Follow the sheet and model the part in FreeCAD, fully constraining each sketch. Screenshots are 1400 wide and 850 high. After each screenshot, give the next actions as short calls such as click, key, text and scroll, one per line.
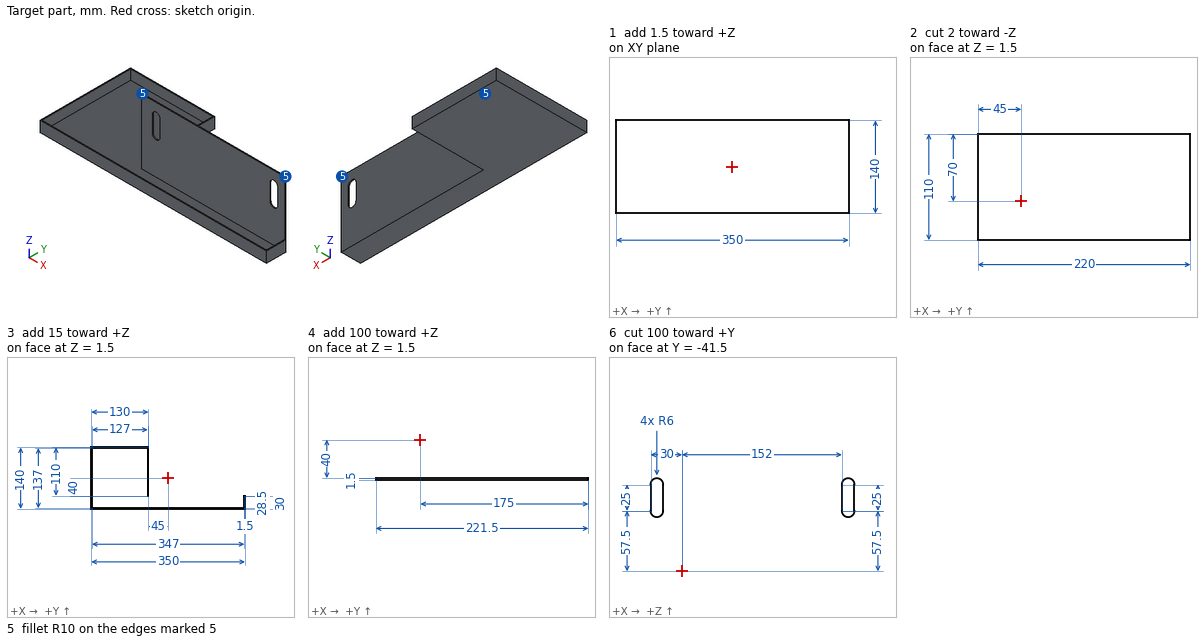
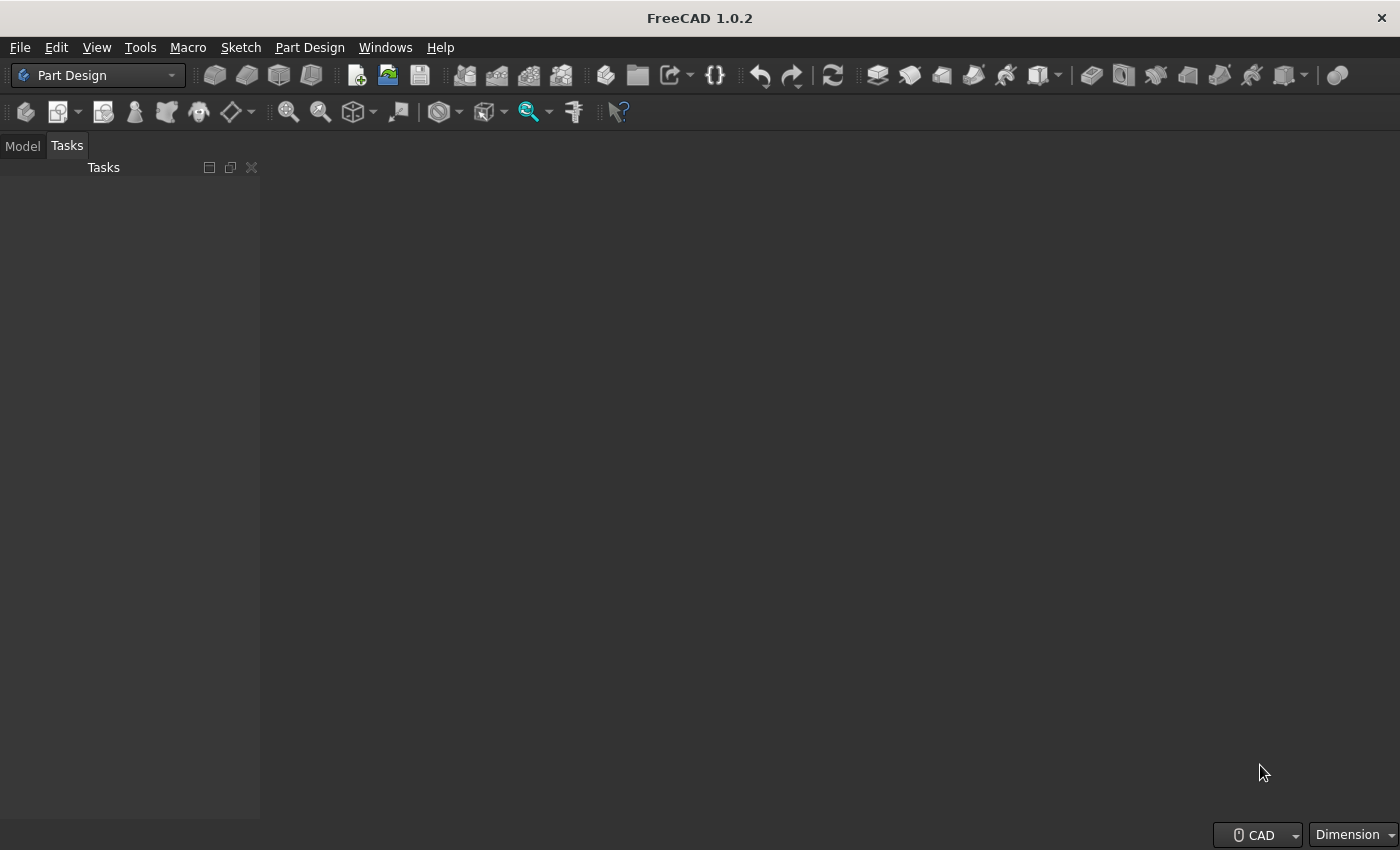
click(356, 76)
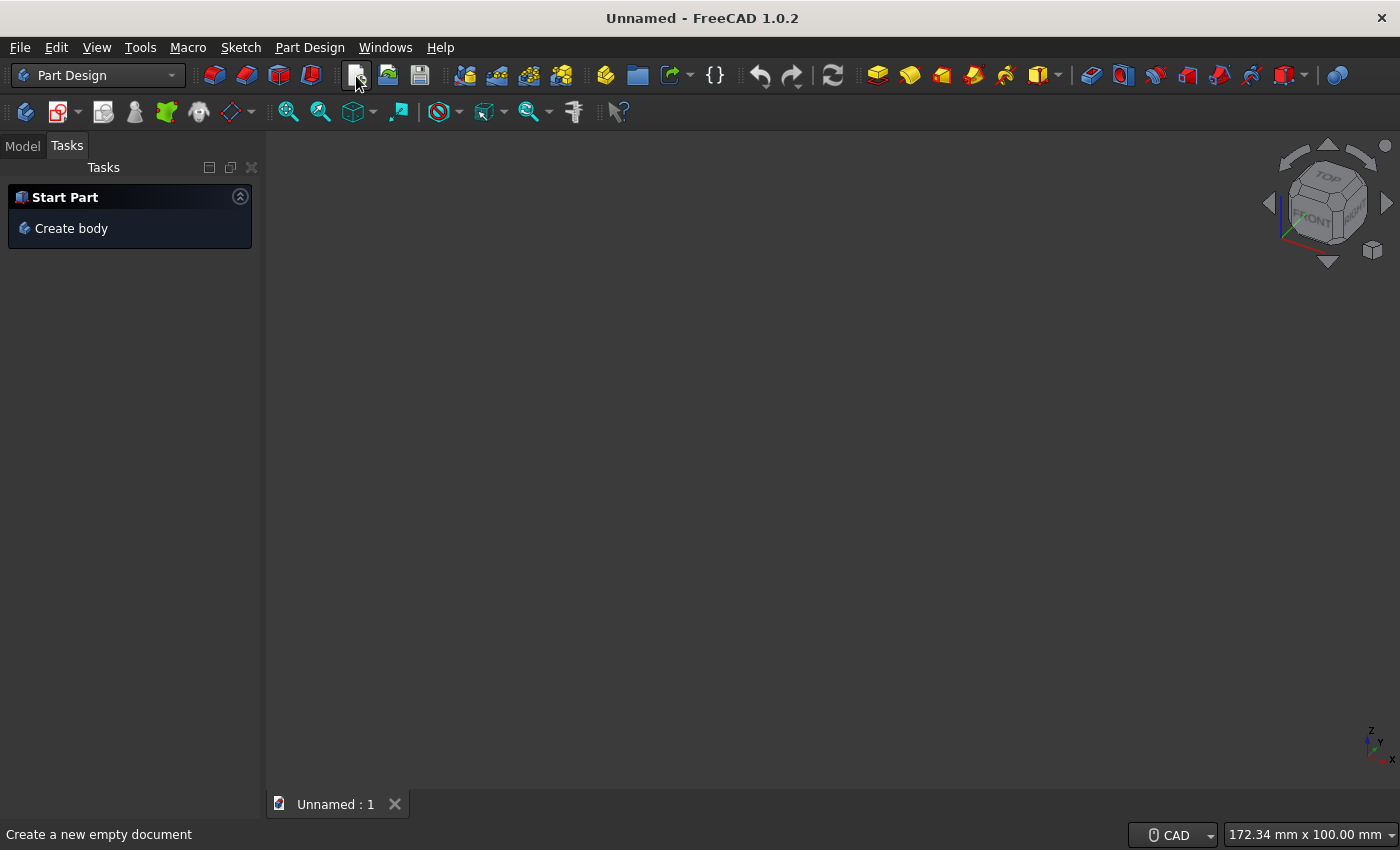
click(58, 112)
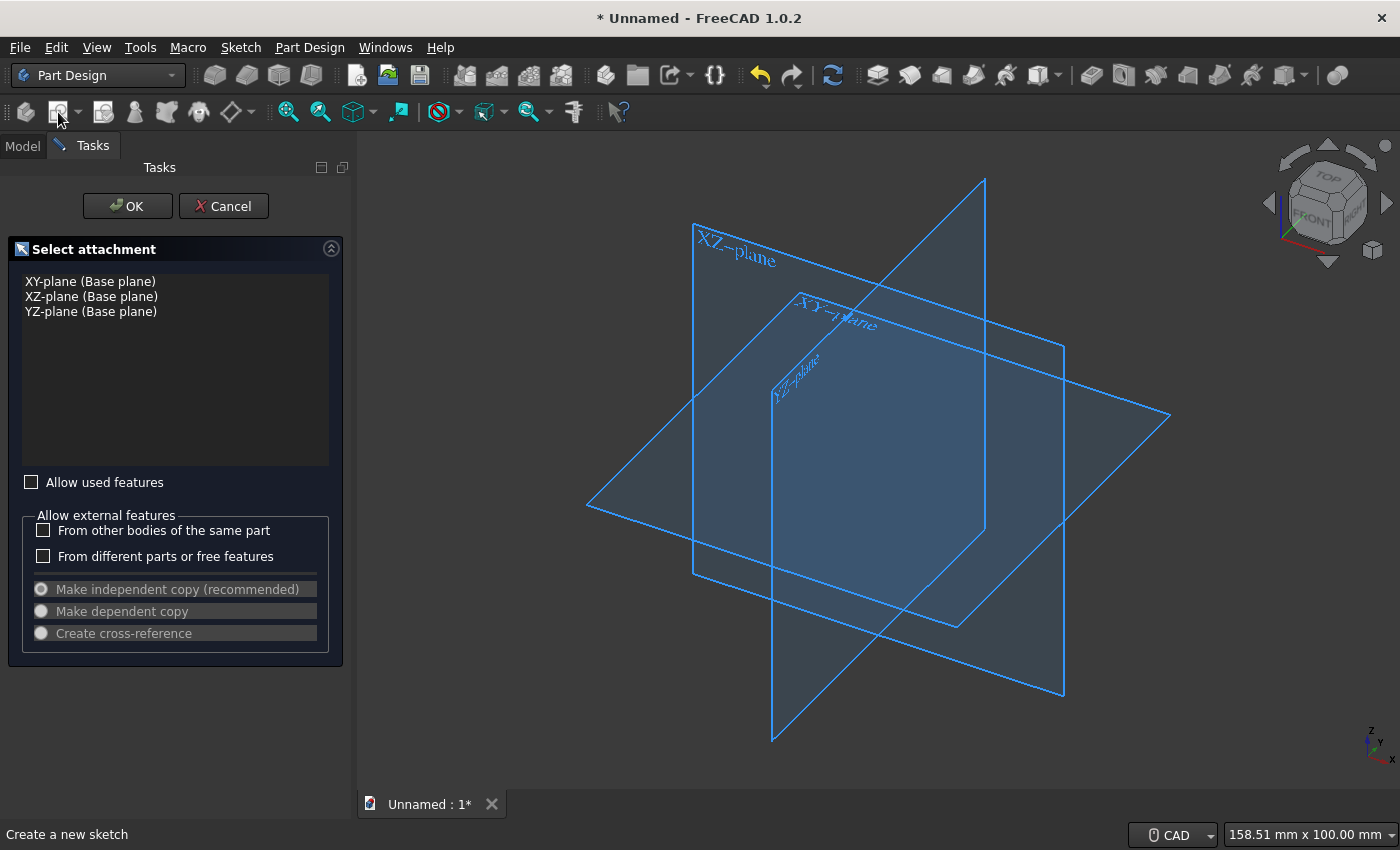
click(82, 282)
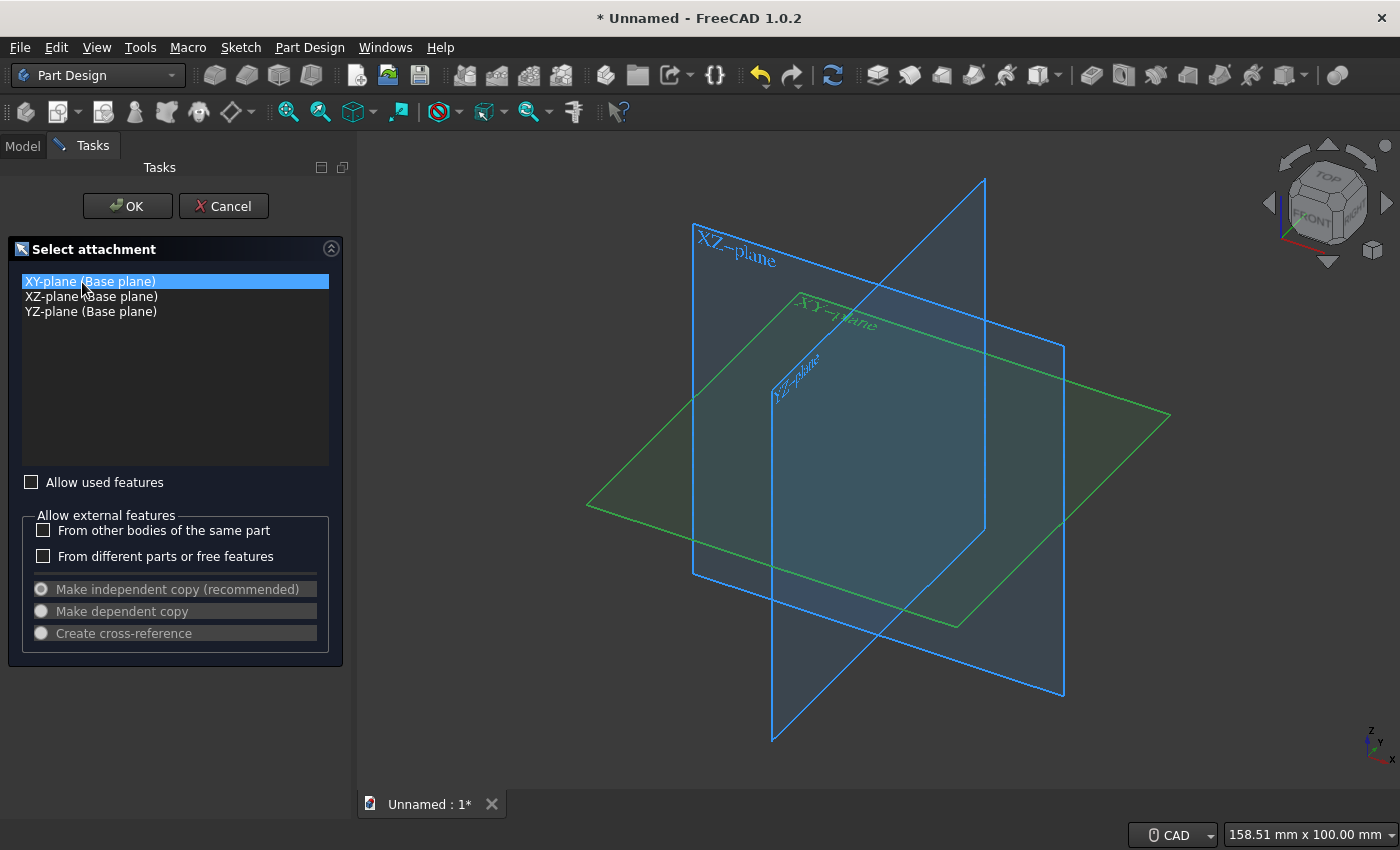
click(128, 206)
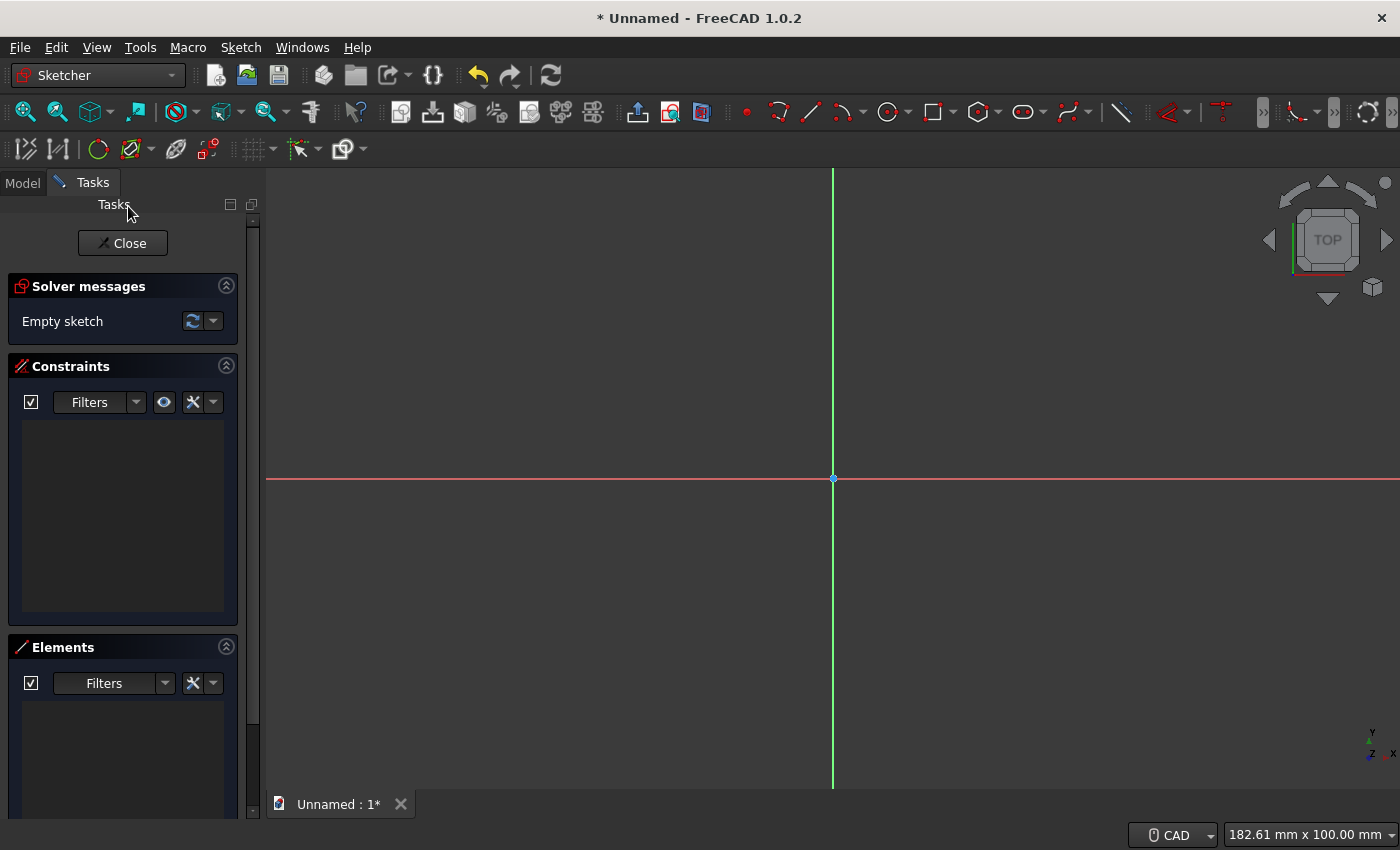
scroll(735, 478, down, 6)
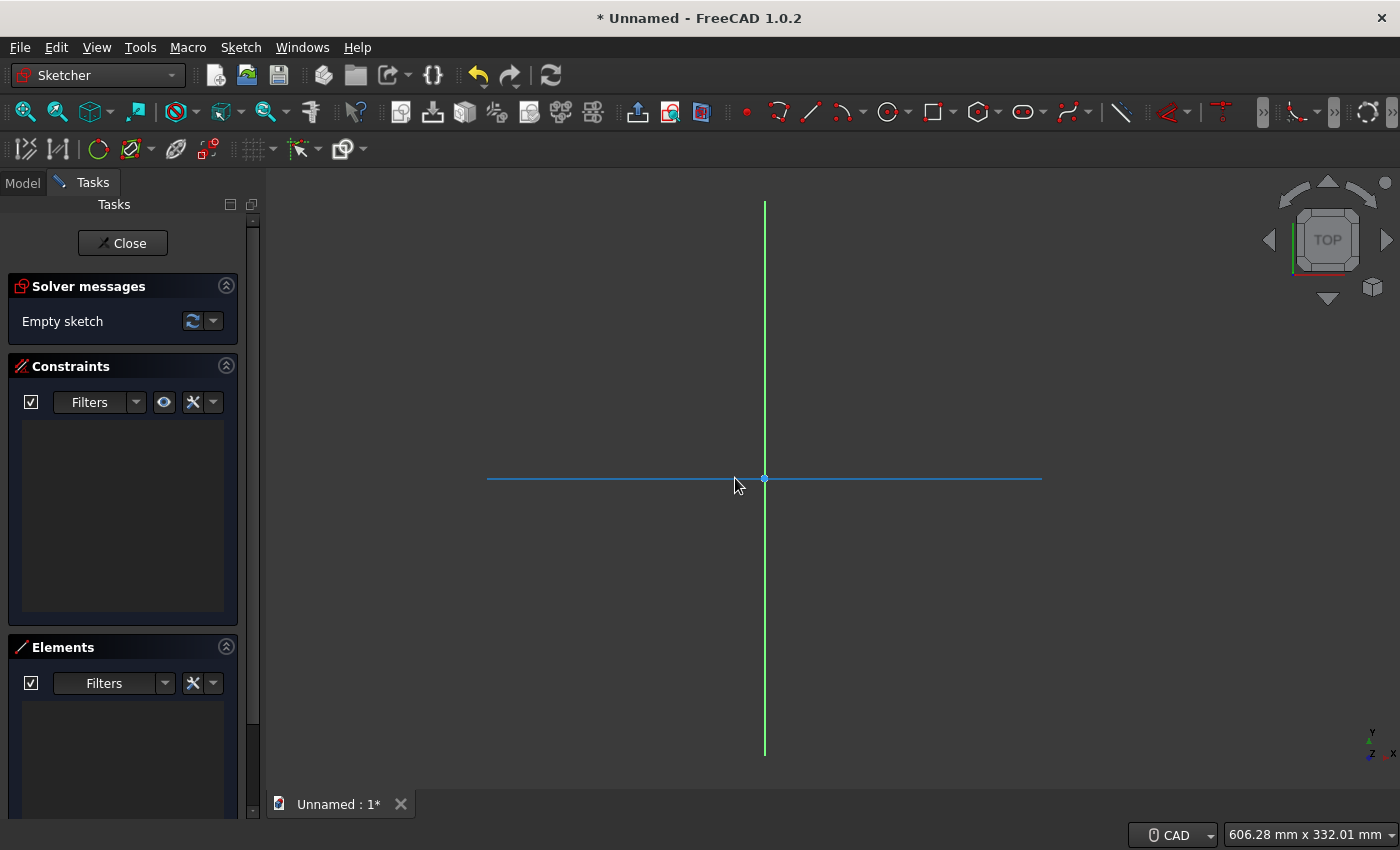
key(g)
key(v)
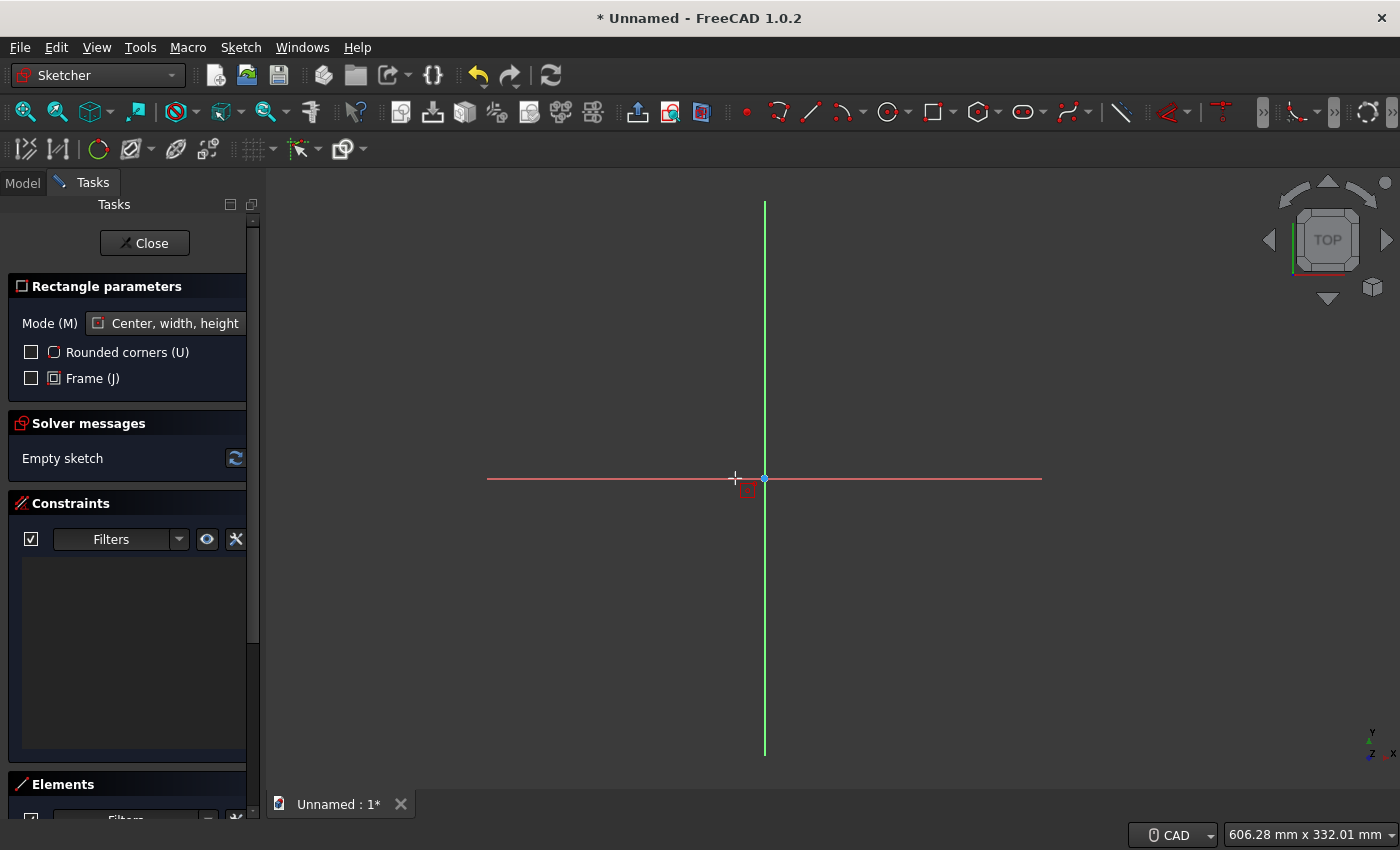
click(765, 478)
click(1092, 348)
key(Escape)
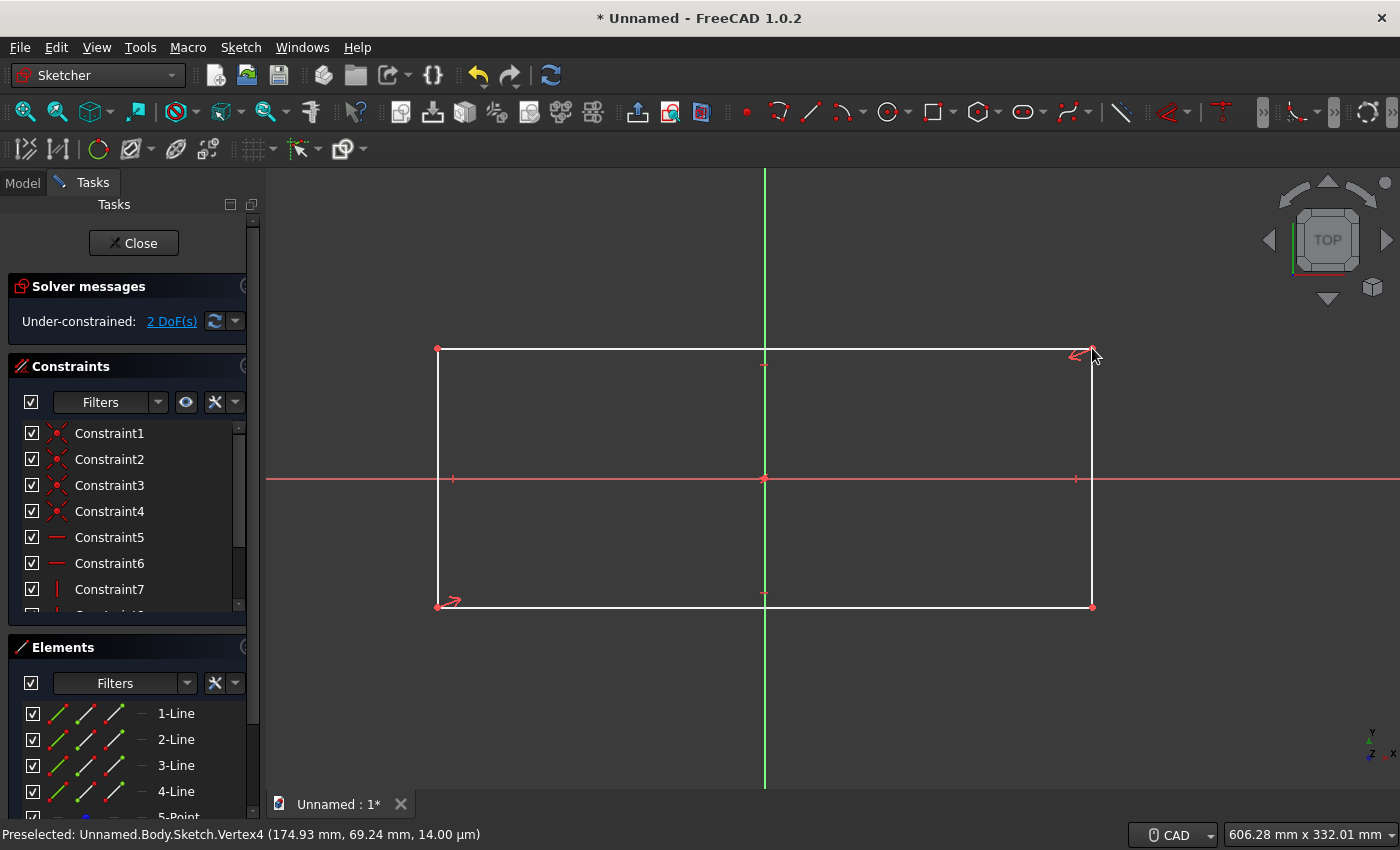
click(1168, 112)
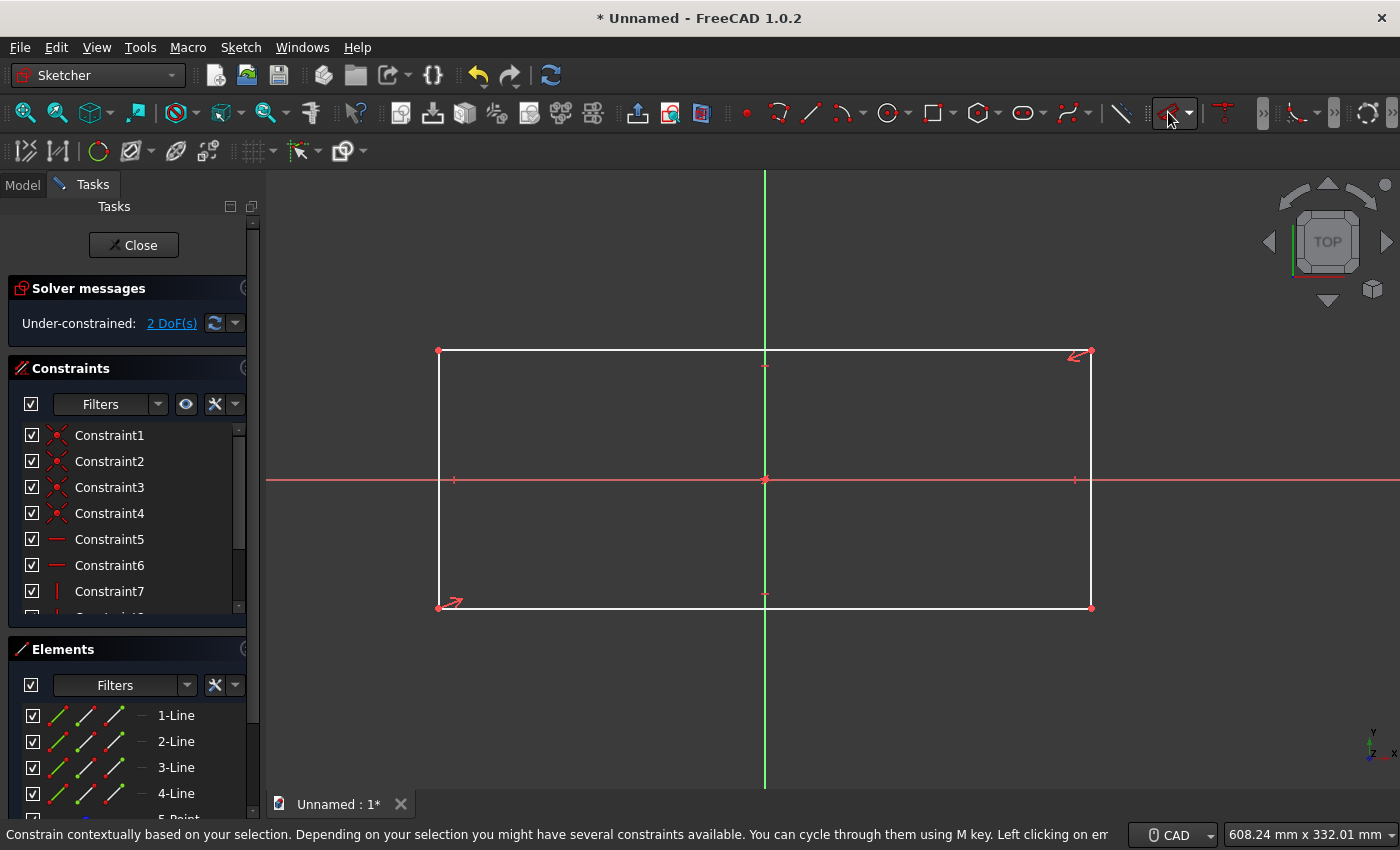
click(635, 609)
click(615, 643)